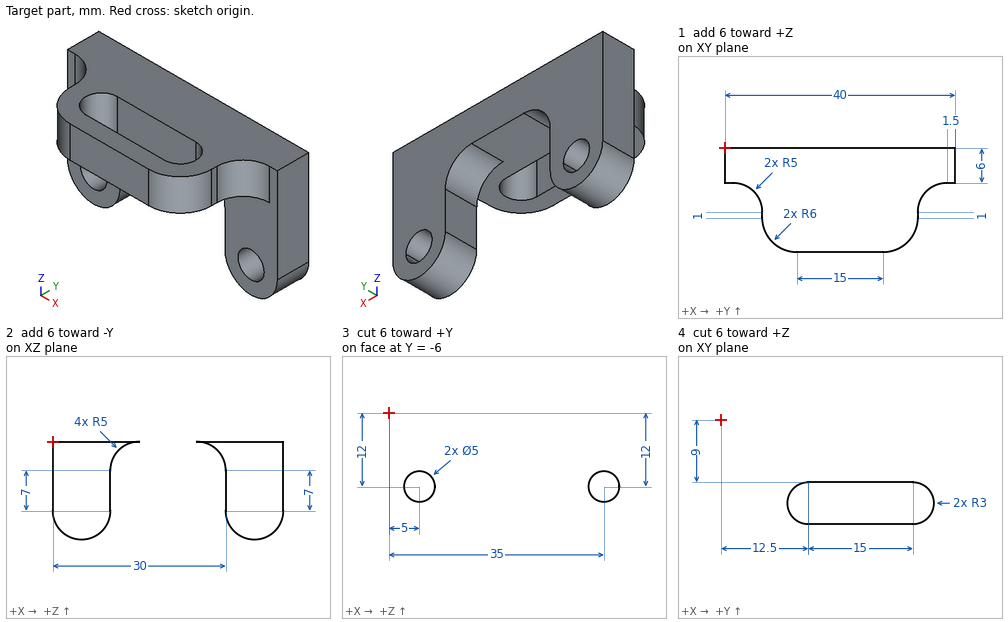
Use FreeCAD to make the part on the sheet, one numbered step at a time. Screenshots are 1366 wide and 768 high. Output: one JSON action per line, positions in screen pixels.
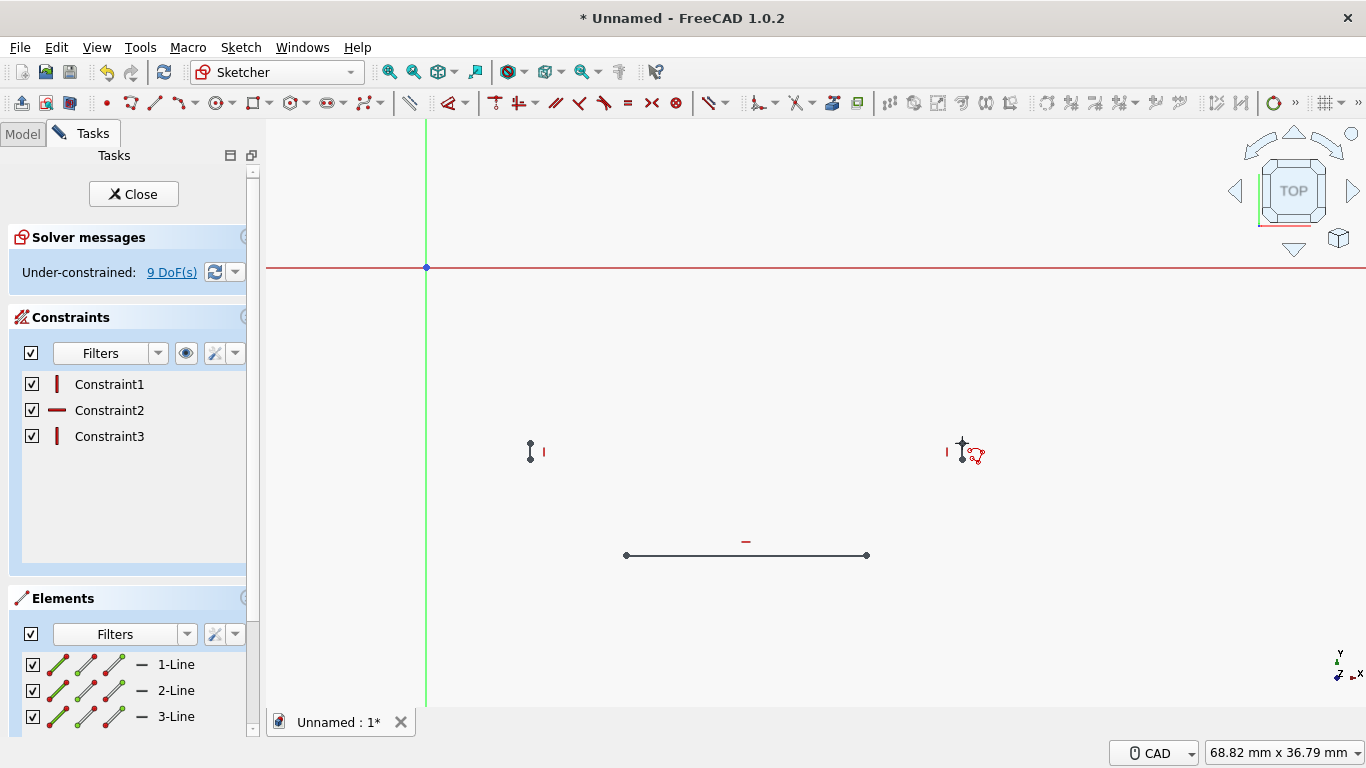
{"action": "left_click", "coordinate": [1042, 363]}
{"action": "left_click", "coordinate": [1066, 363]}
{"action": "left_click", "coordinate": [1066, 268]}
{"action": "left_click", "coordinate": [426, 268]}
{"action": "left_click", "coordinate": [435, 363]}
{"action": "left_click", "coordinate": [450, 363]}
{"action": "right_click", "coordinate": [450, 363]}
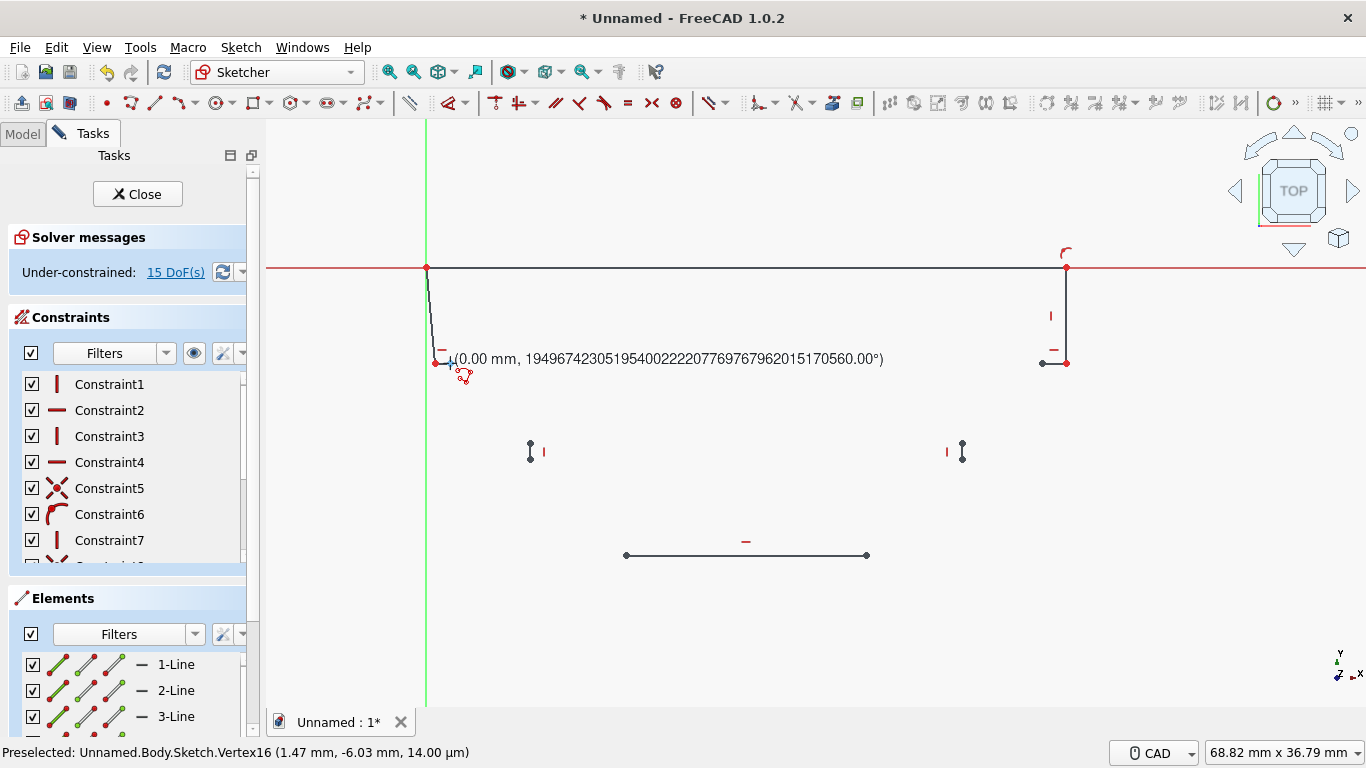
{"action": "left_click", "coordinate": [180, 104]}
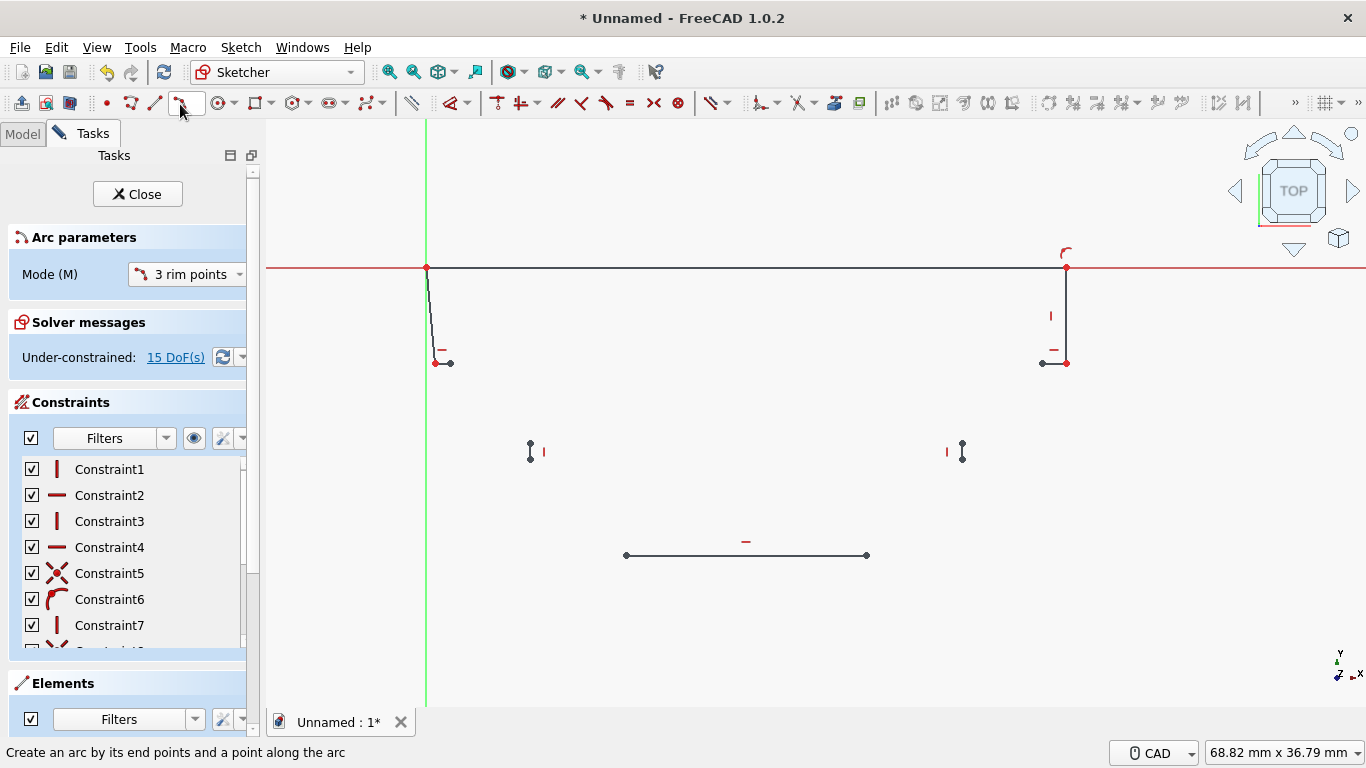
{"action": "scroll", "coordinate": [530, 459], "scroll_direction": "up", "scroll_amount": 4}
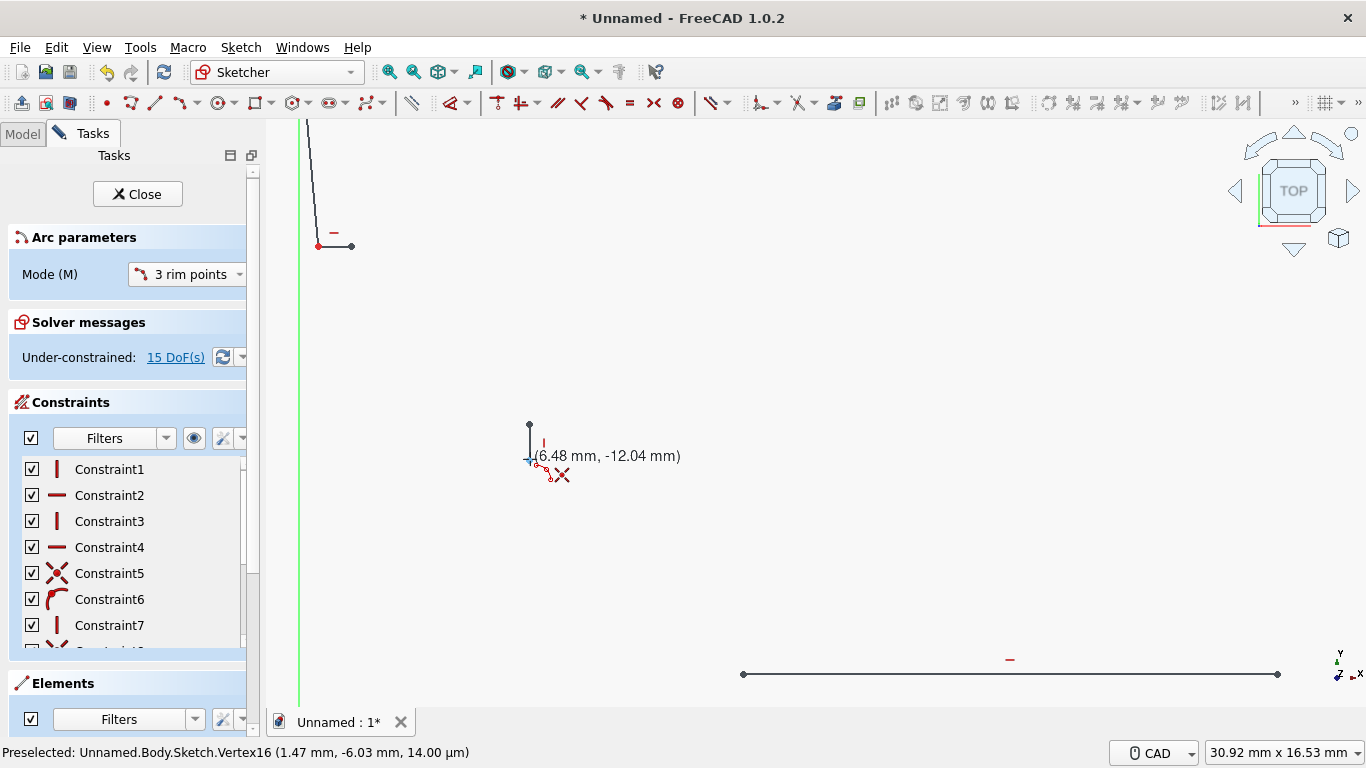
{"action": "left_click", "coordinate": [530, 461]}
{"action": "left_click", "coordinate": [743, 674]}
{"action": "left_click", "coordinate": [593, 610]}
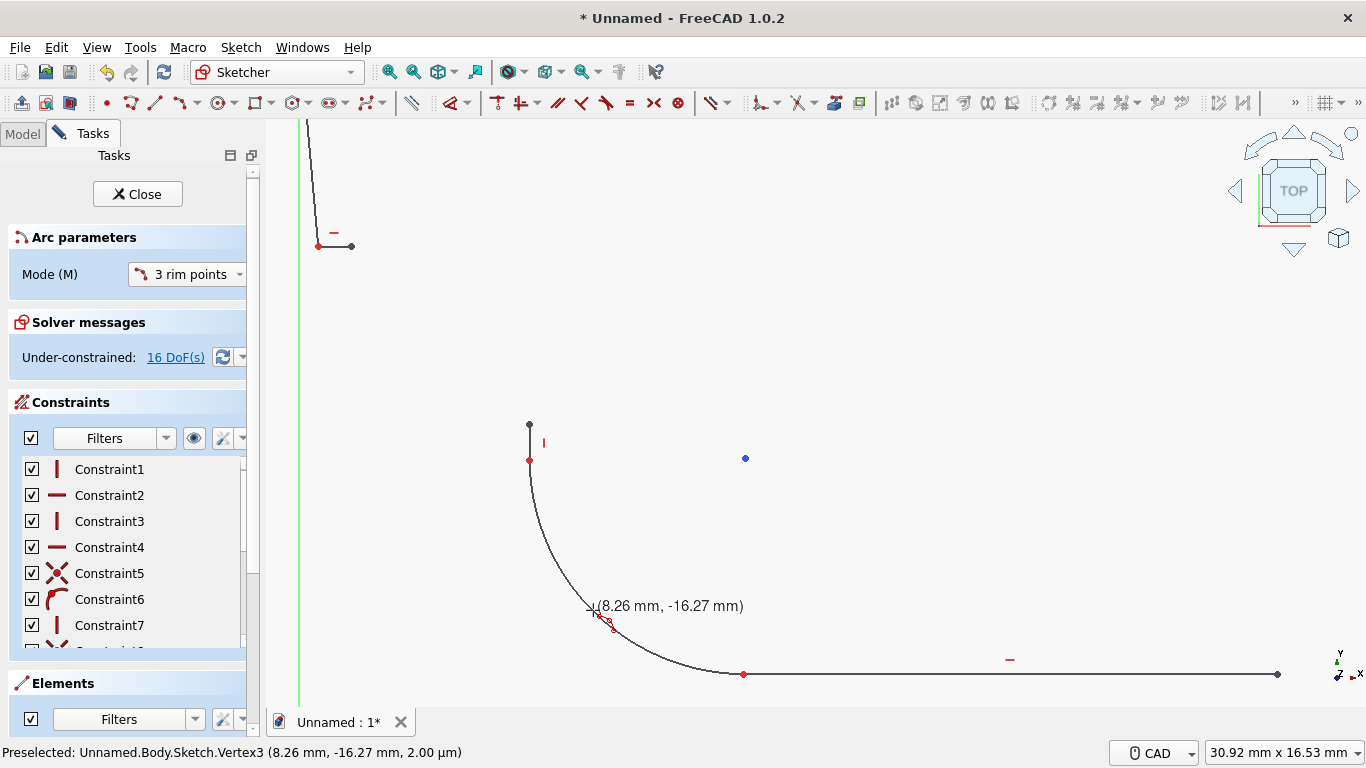
{"action": "scroll", "coordinate": [533, 462], "scroll_direction": "down", "scroll_amount": 4}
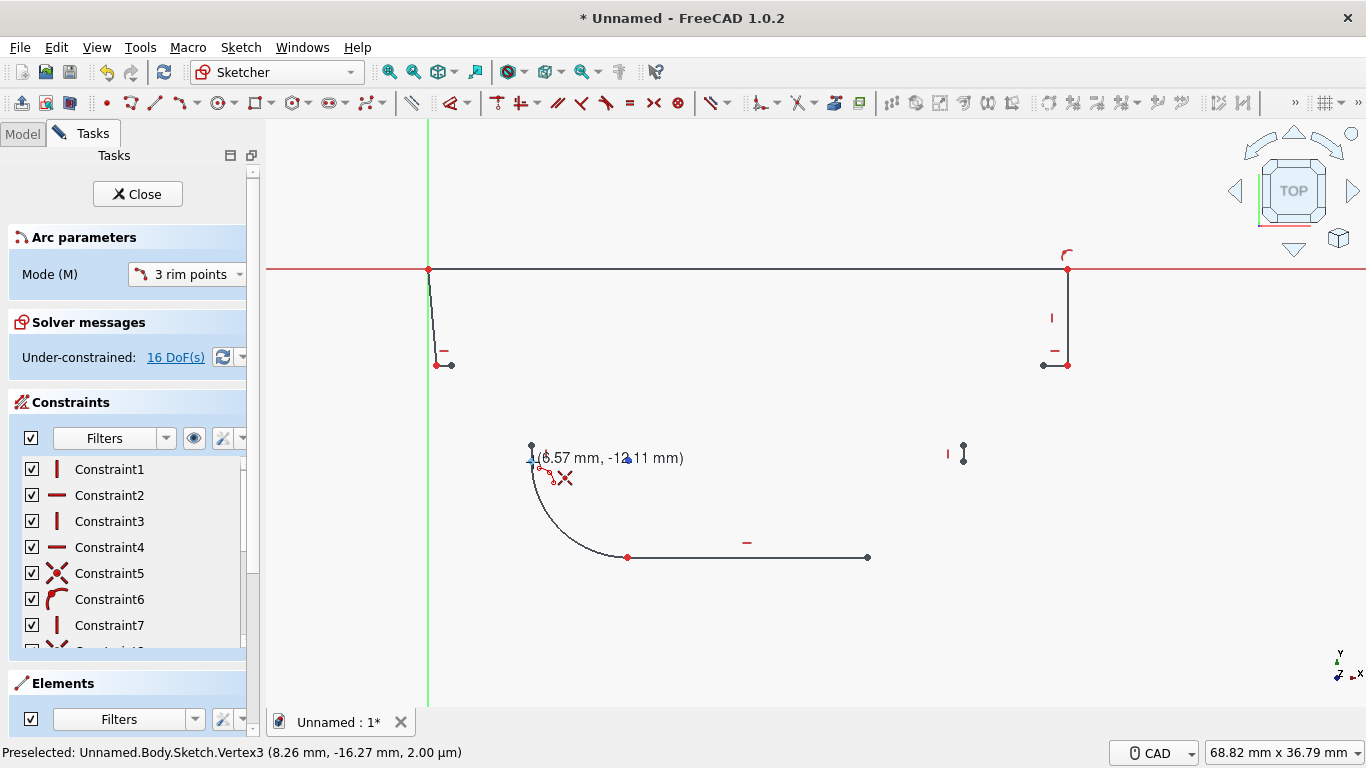
{"action": "left_click", "coordinate": [868, 558]}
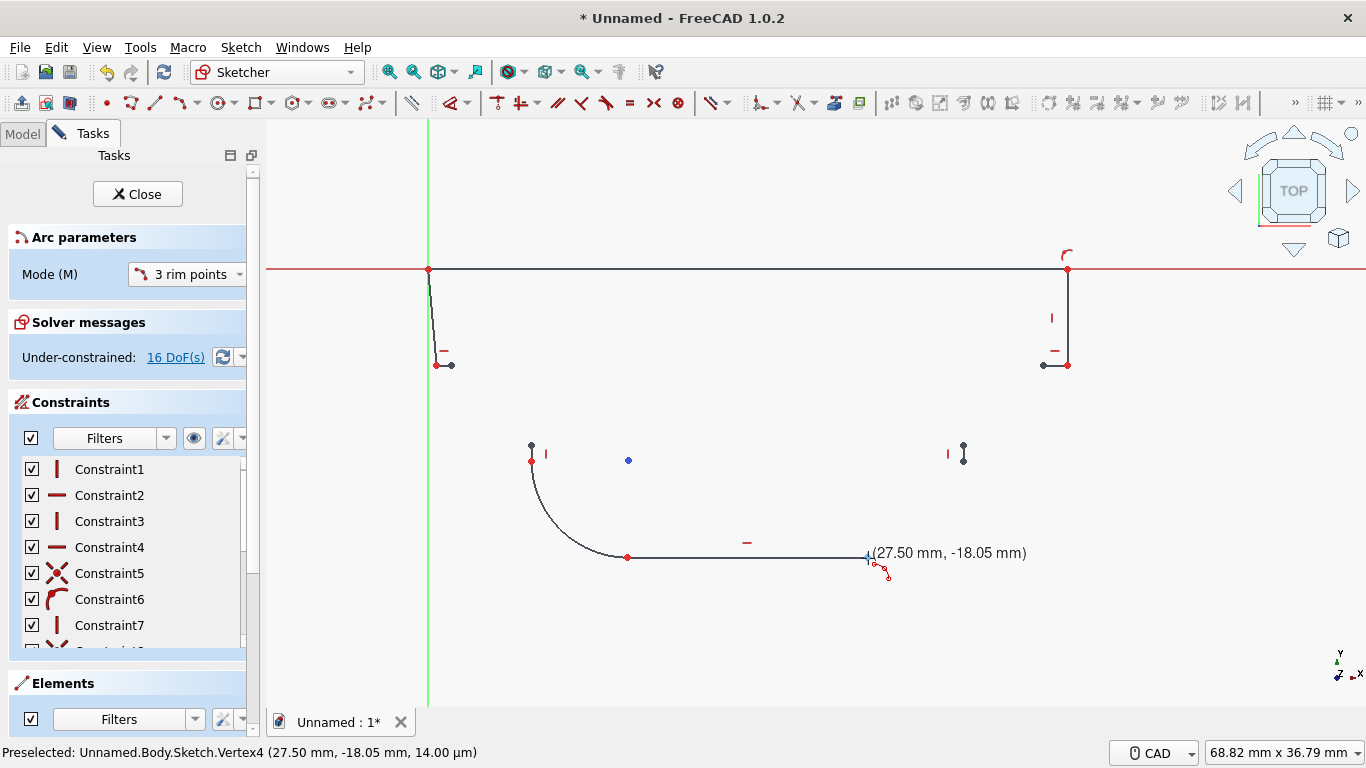
{"action": "scroll", "coordinate": [964, 461], "scroll_direction": "up", "scroll_amount": 4}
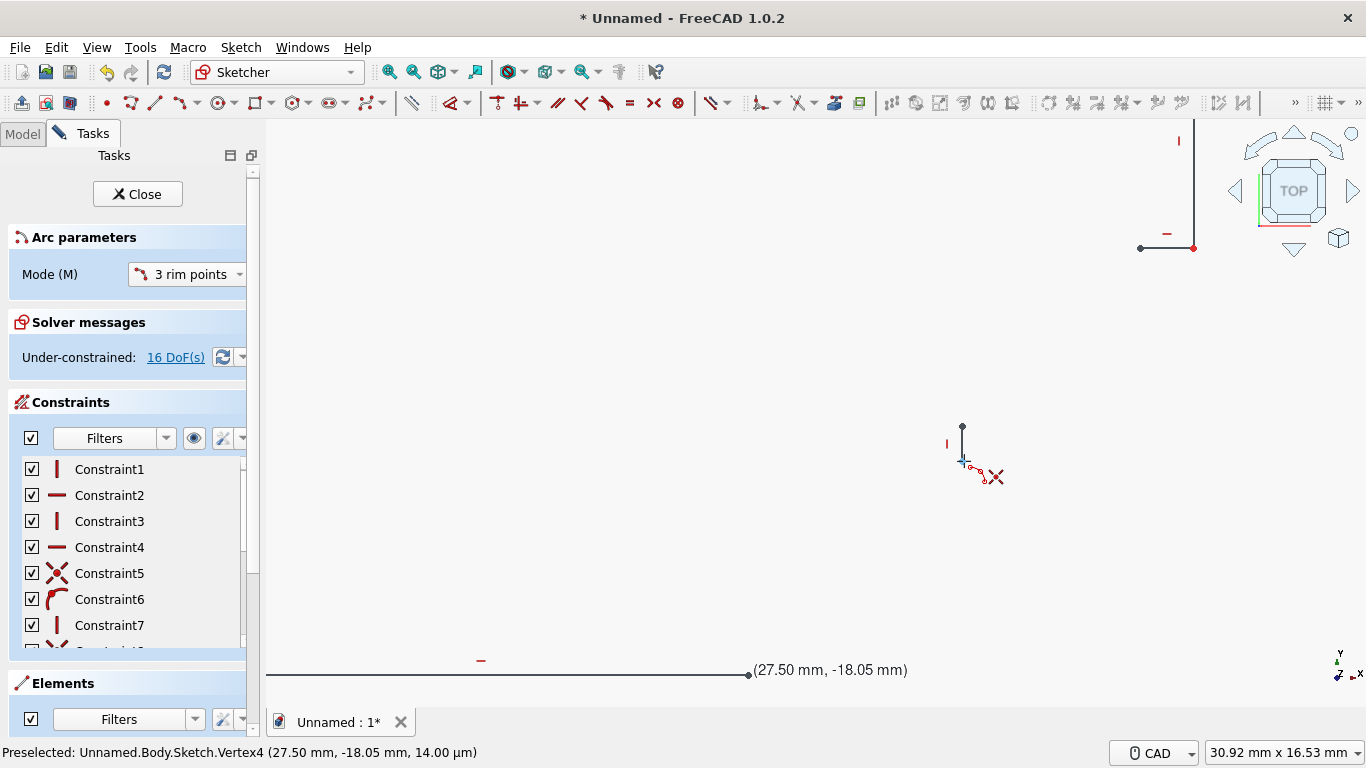
{"action": "left_click", "coordinate": [962, 462]}
{"action": "left_click", "coordinate": [900, 611]}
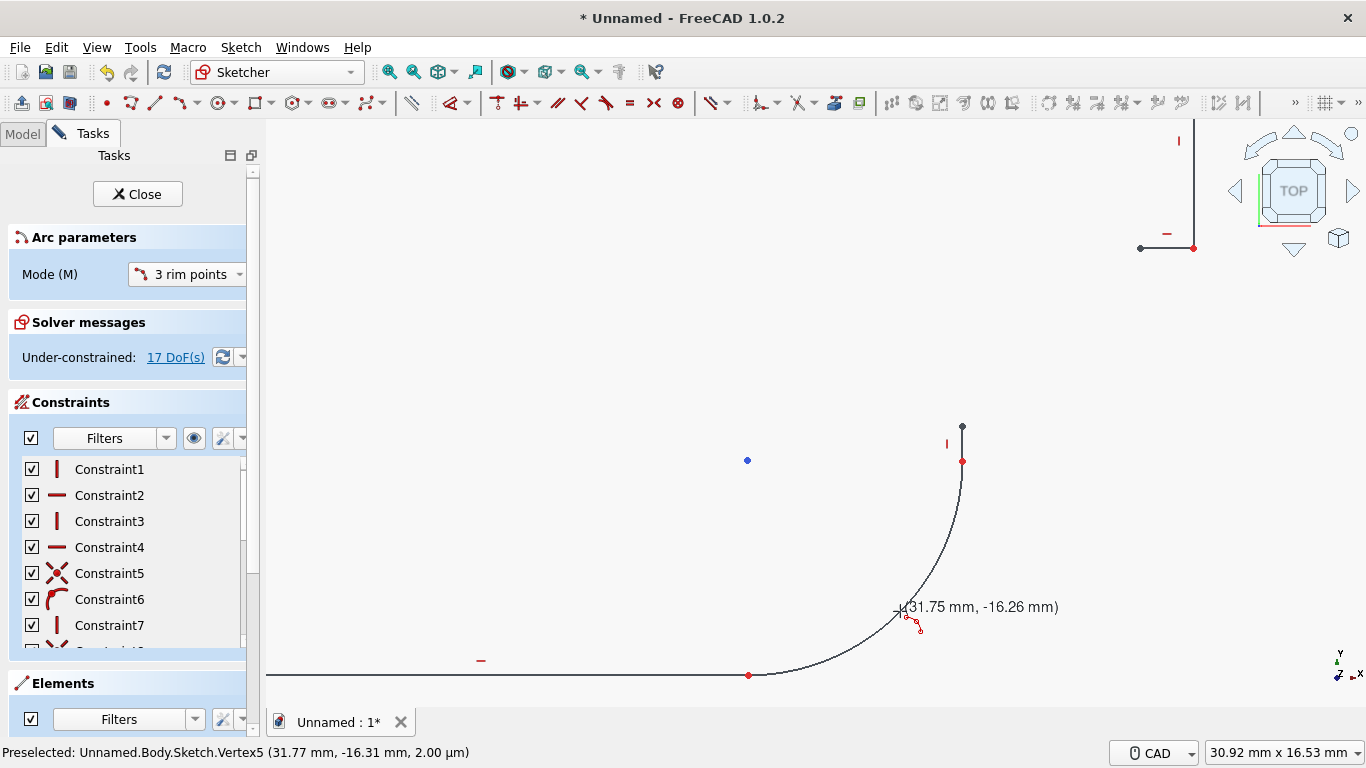
{"action": "left_click", "coordinate": [962, 426]}
{"action": "left_click", "coordinate": [1140, 248]}
{"action": "left_click", "coordinate": [1014, 299]}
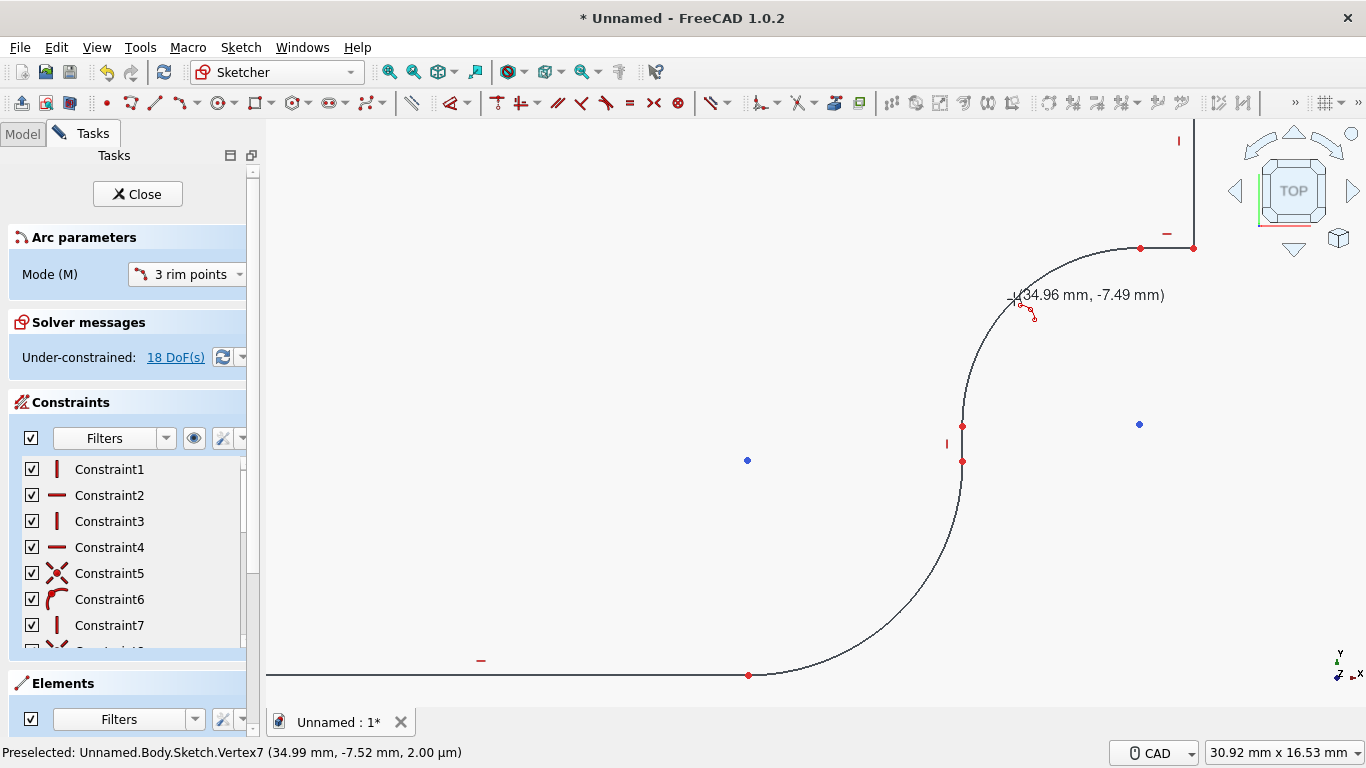
{"action": "scroll", "coordinate": [964, 461], "scroll_direction": "down", "scroll_amount": 4}